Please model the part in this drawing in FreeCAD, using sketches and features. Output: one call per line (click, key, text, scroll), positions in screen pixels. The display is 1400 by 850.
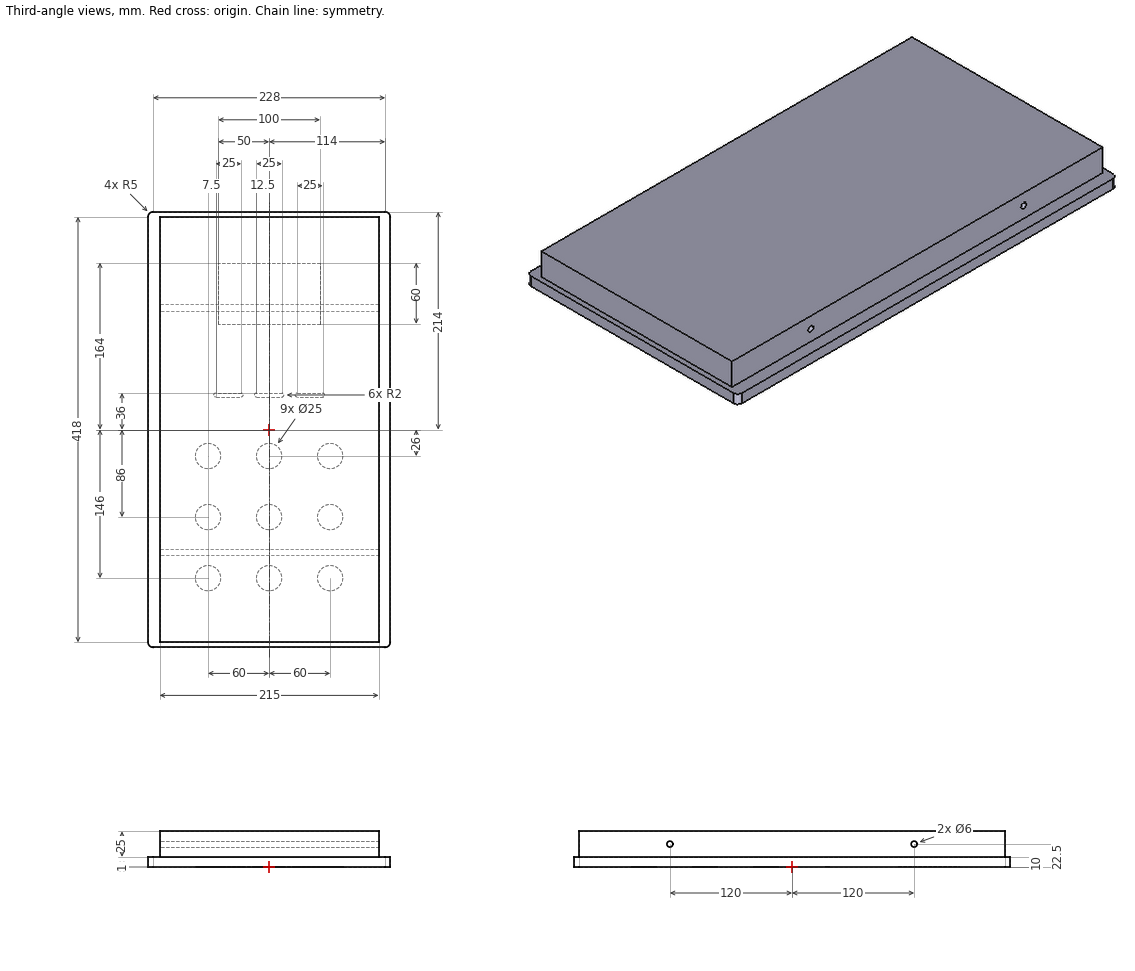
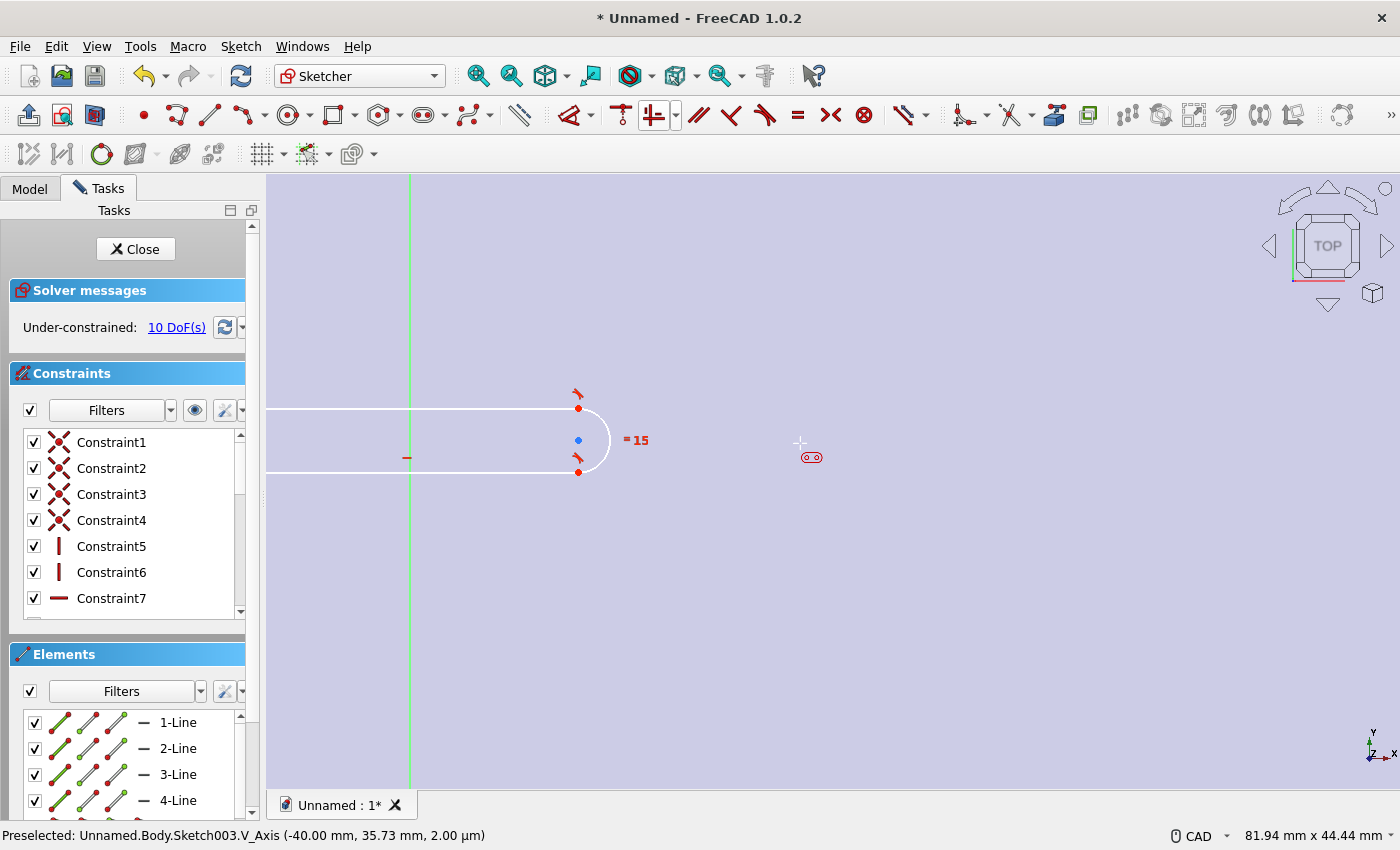
scroll(800, 443, down, 12)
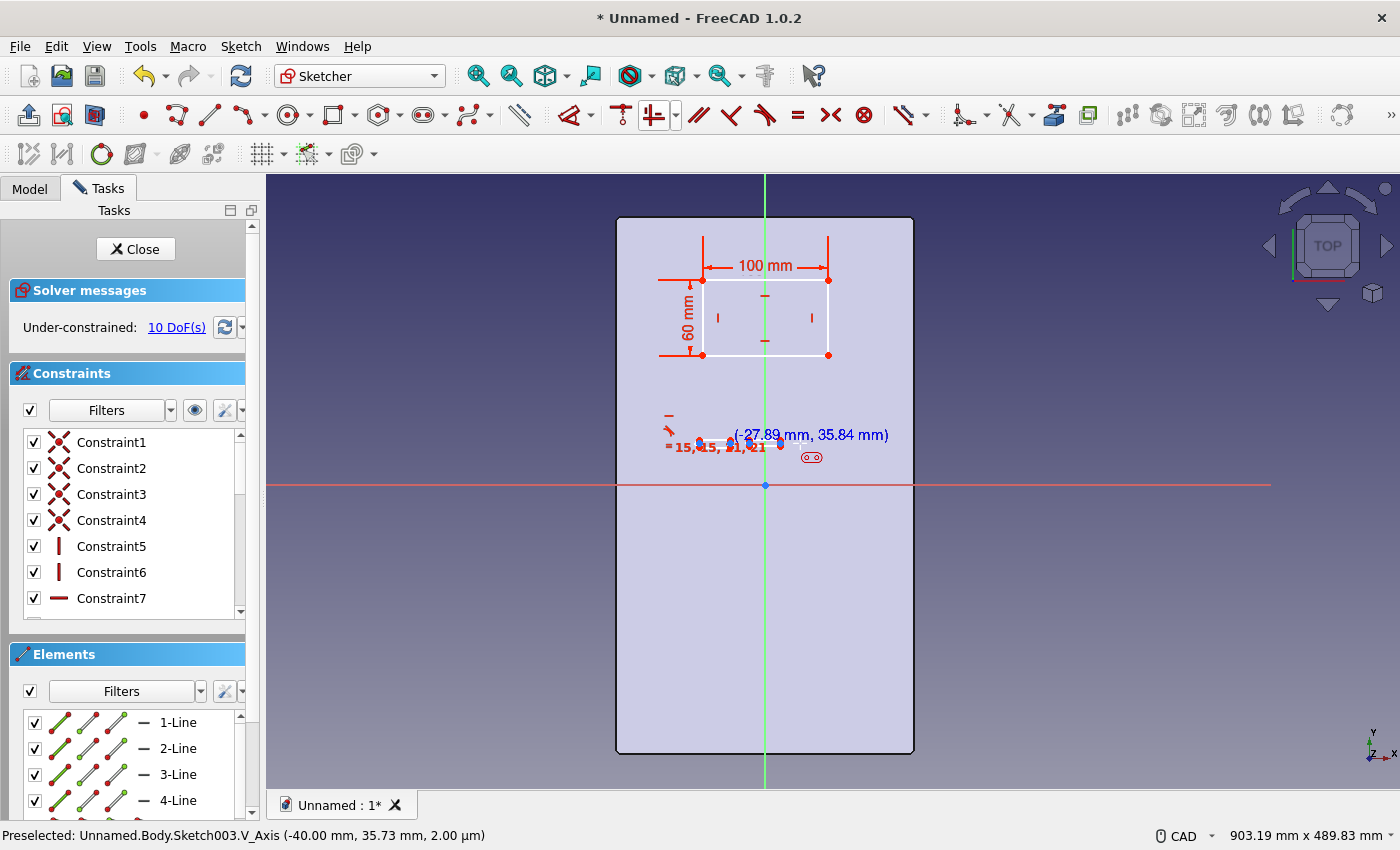
click(800, 443)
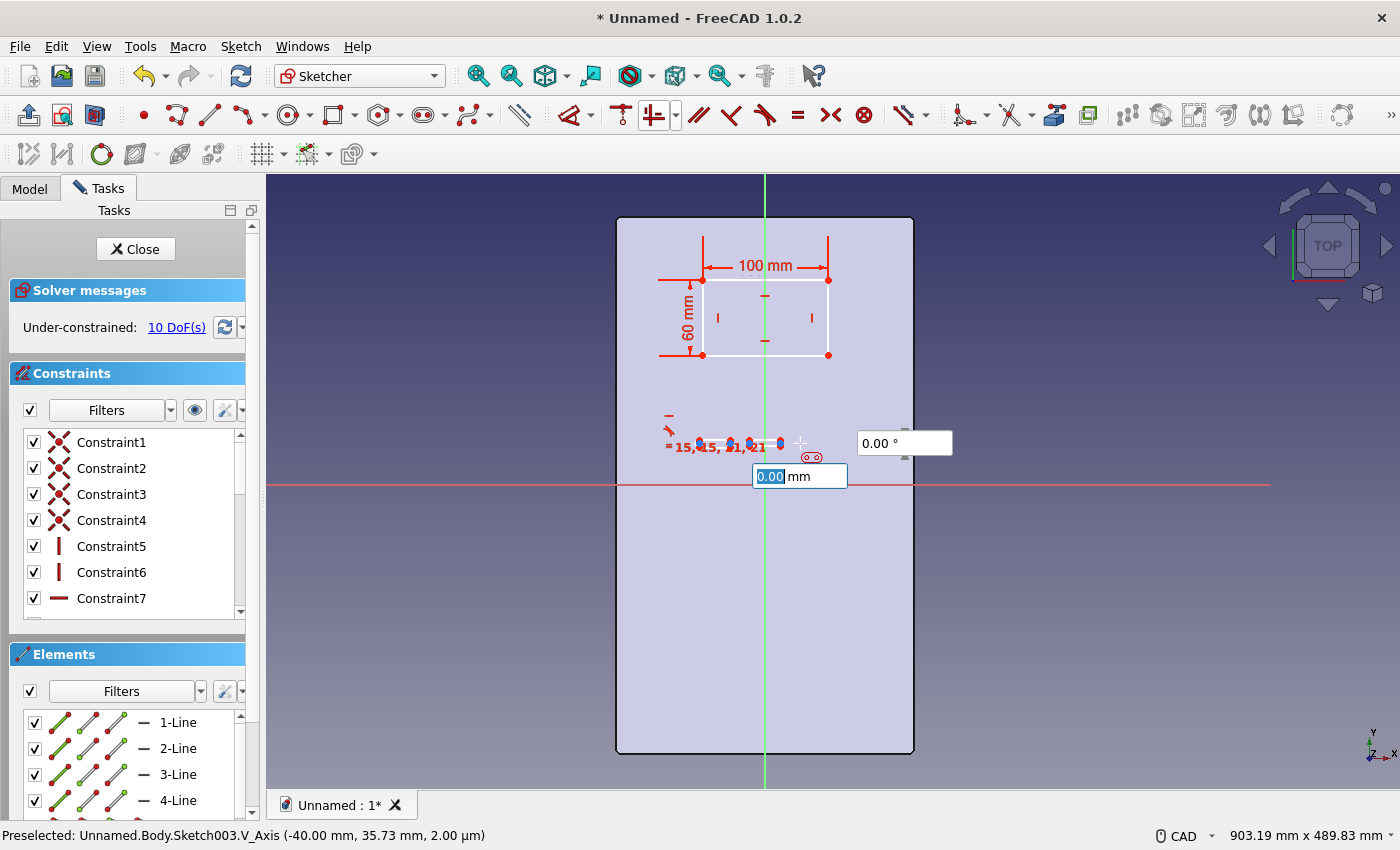
click(831, 443)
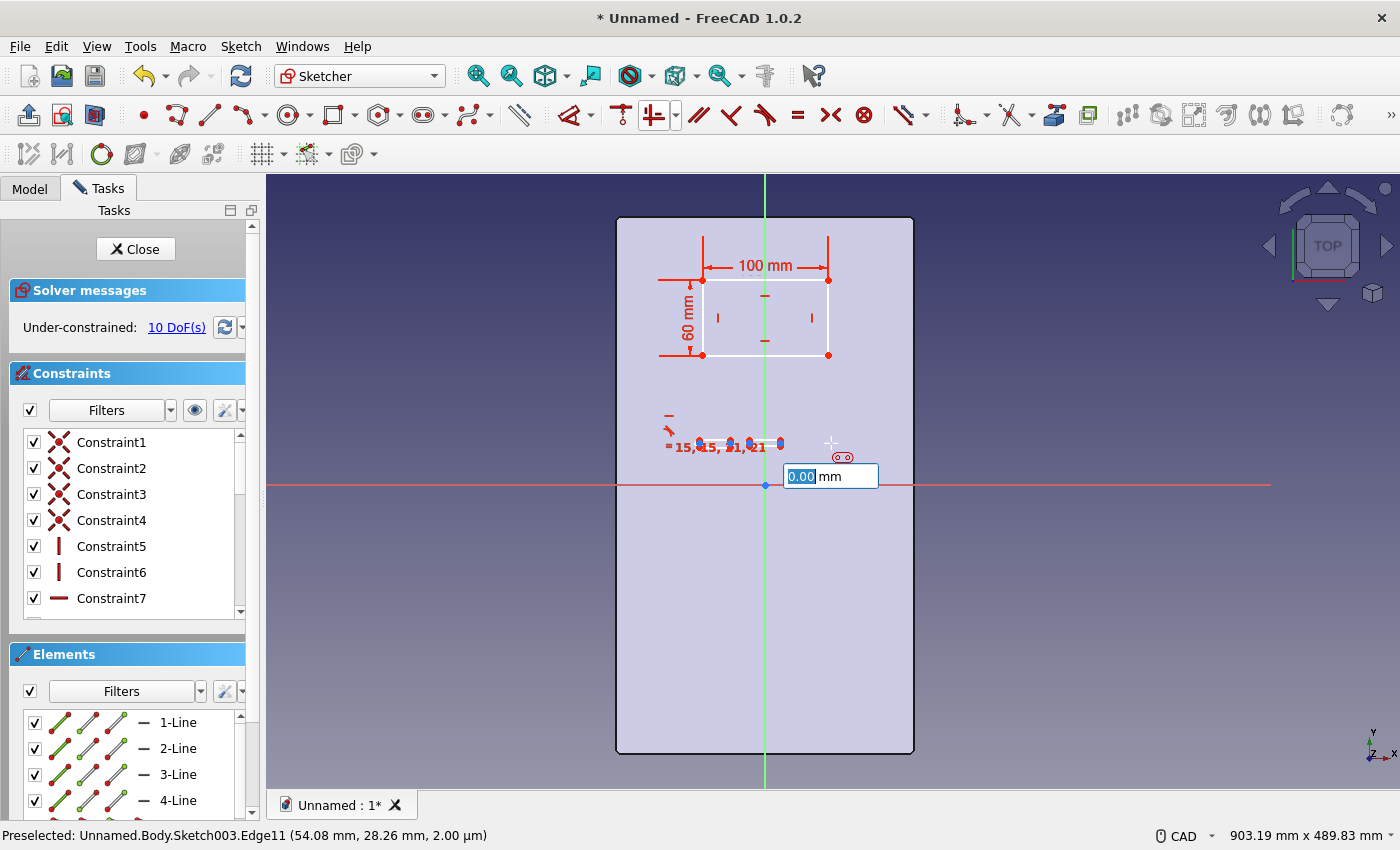
scroll(815, 440, up, 10)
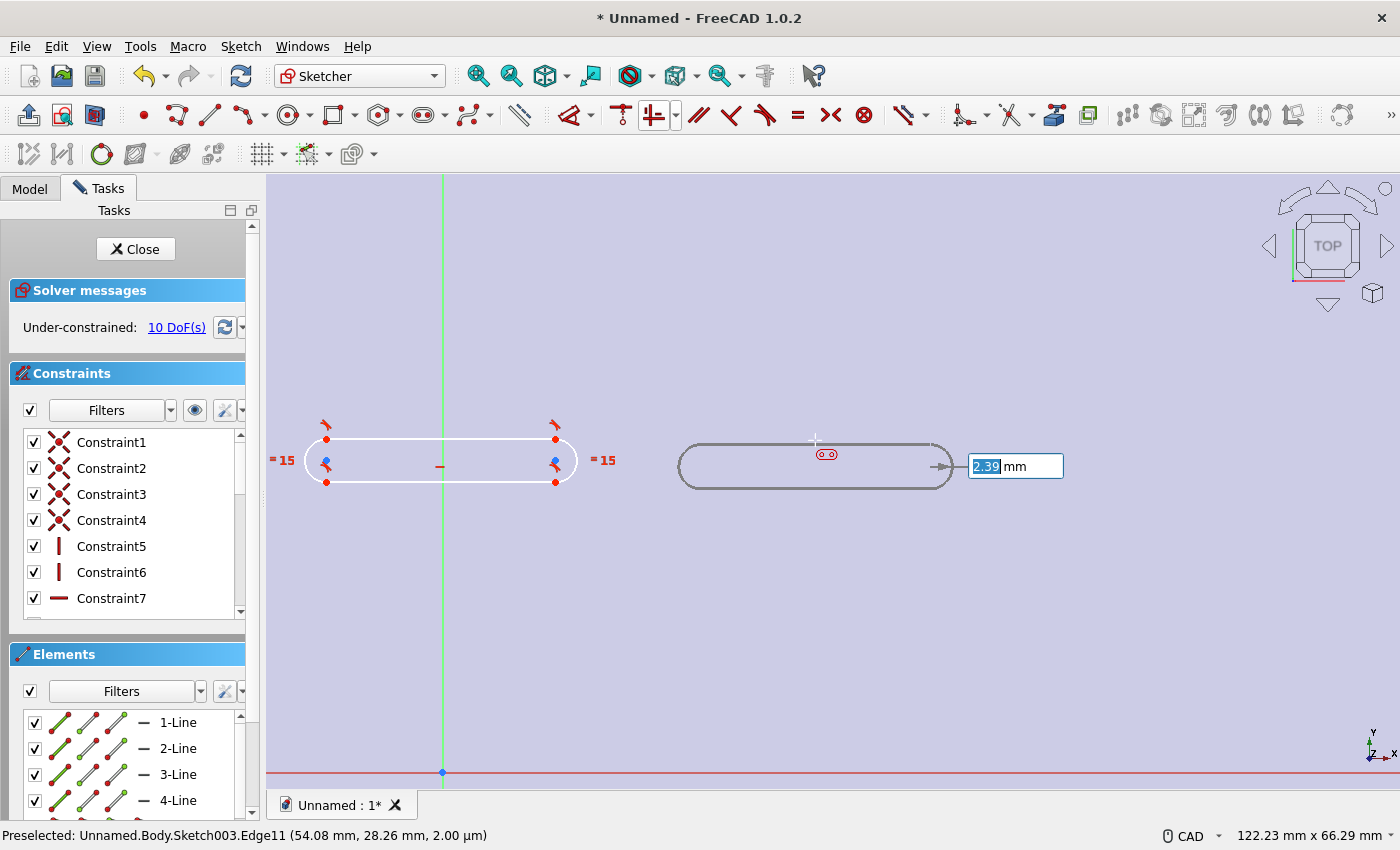
click(814, 439)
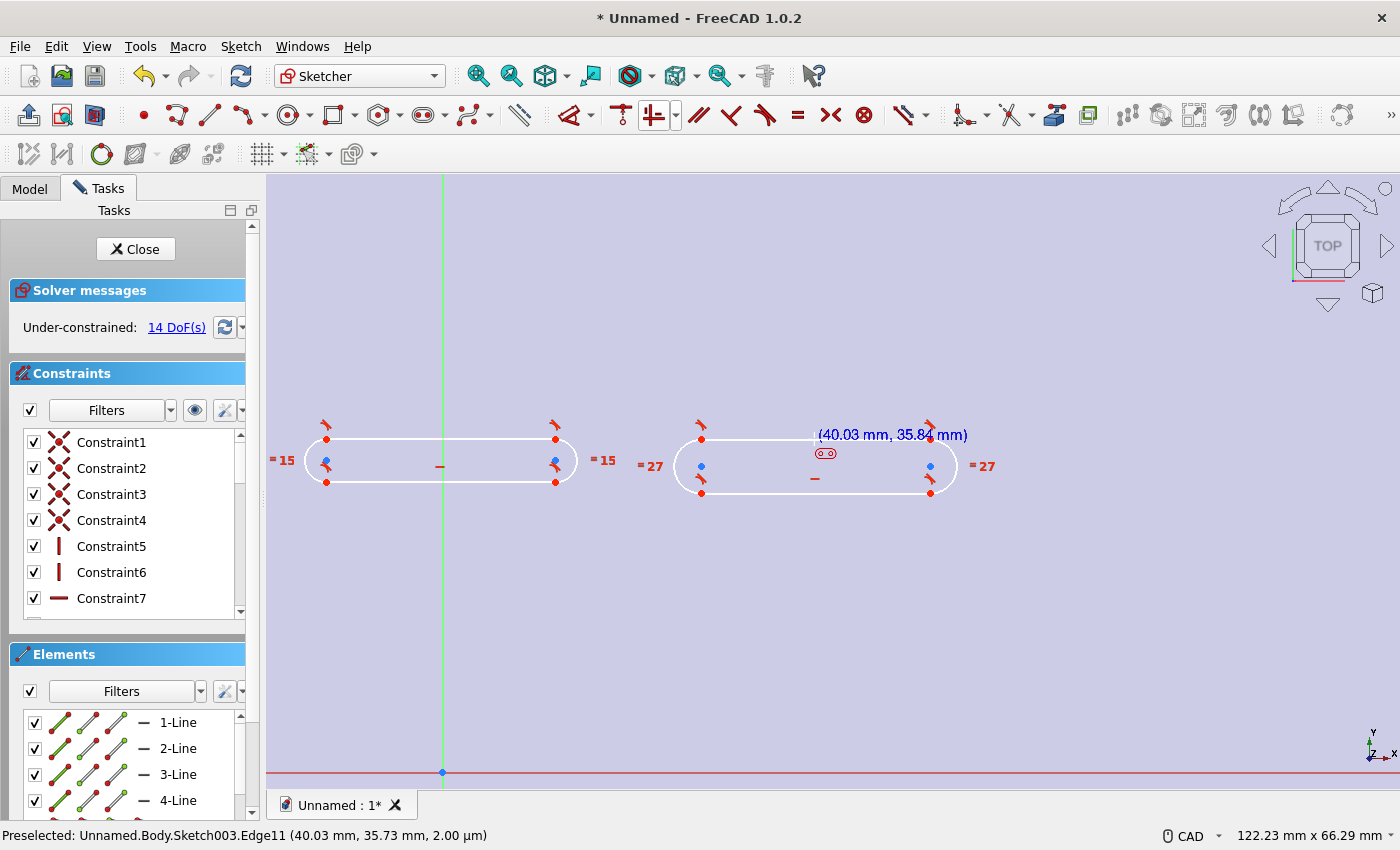
click(288, 116)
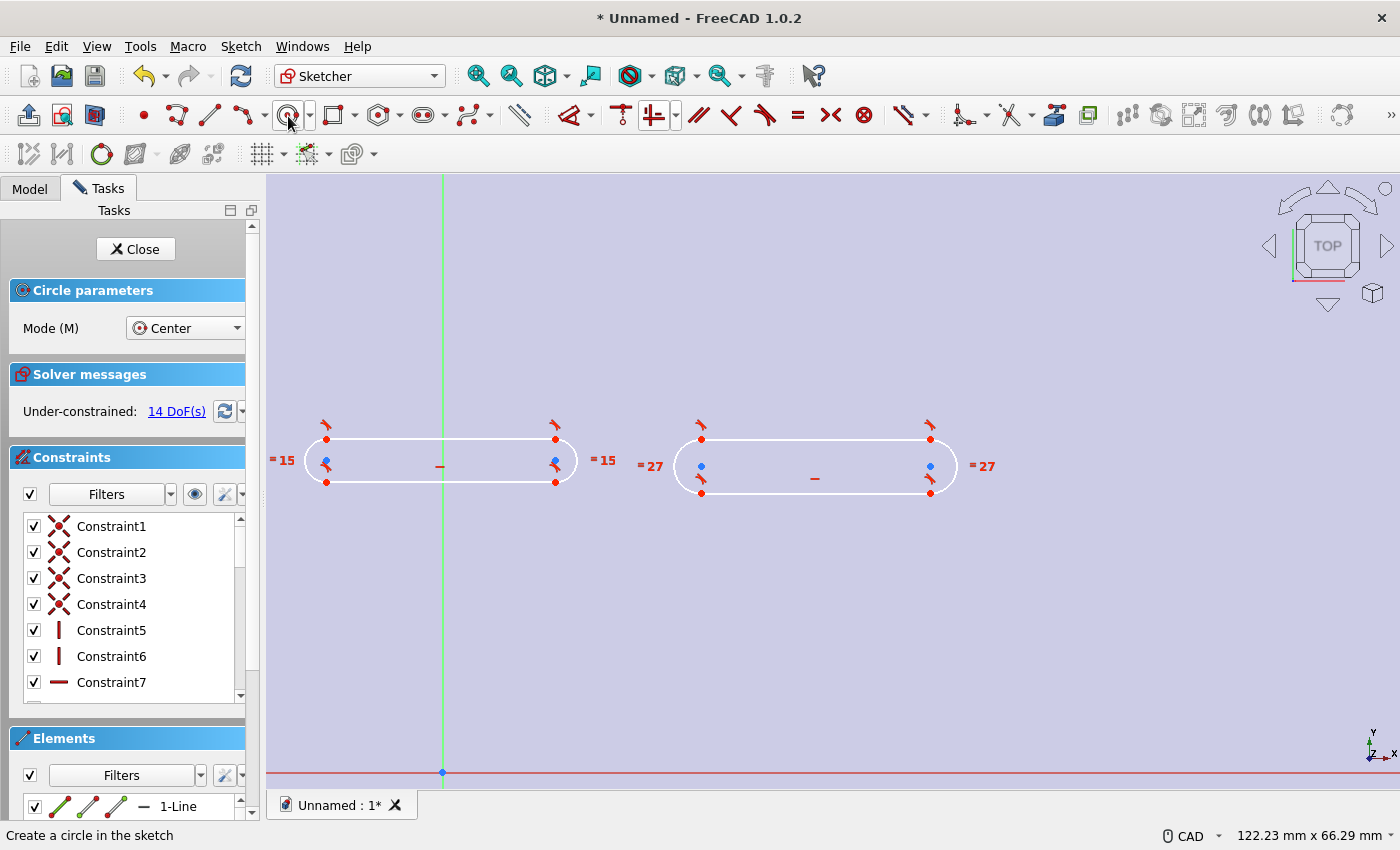
scroll(815, 440, down, 10)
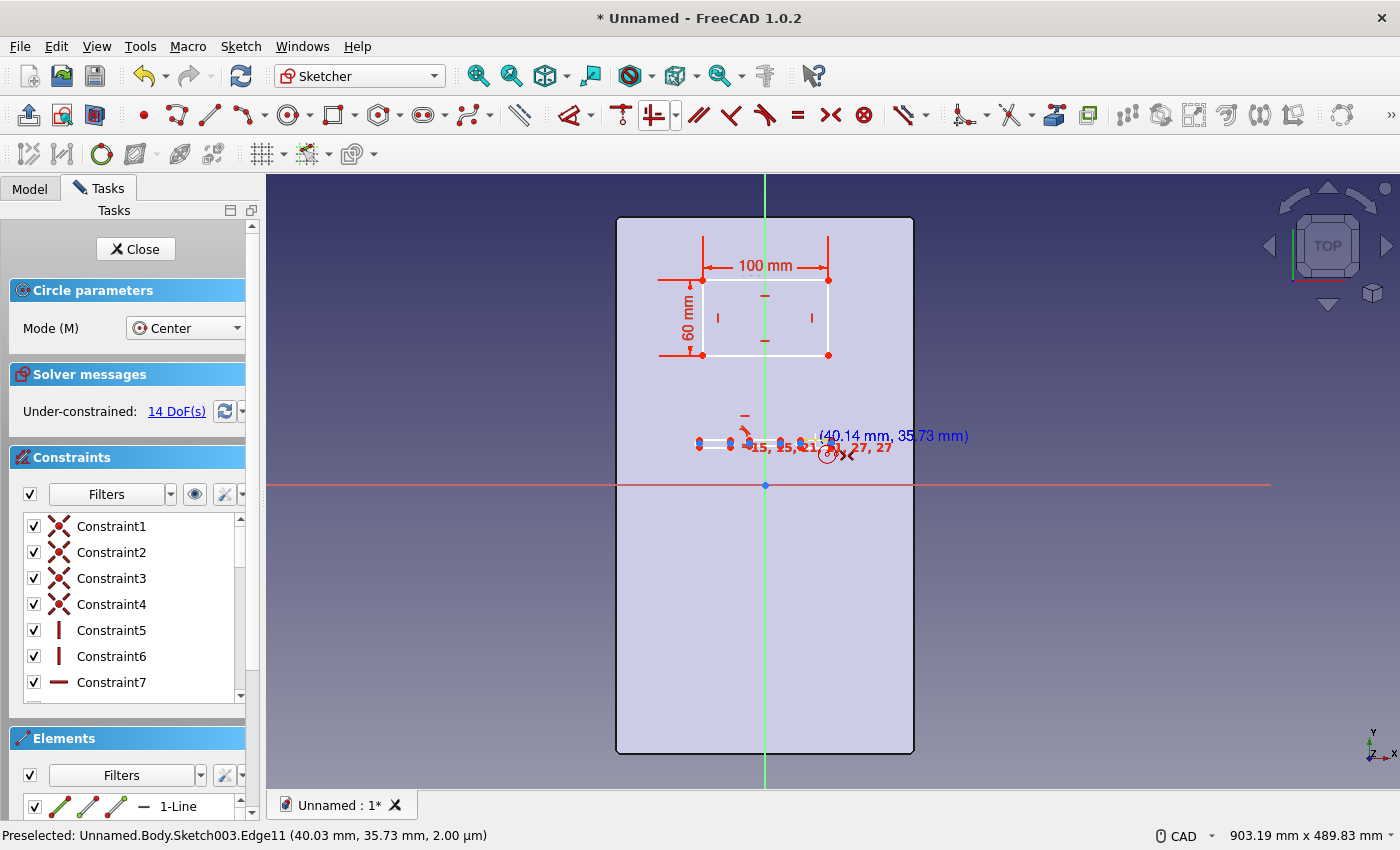
scroll(765, 518, up, 2)